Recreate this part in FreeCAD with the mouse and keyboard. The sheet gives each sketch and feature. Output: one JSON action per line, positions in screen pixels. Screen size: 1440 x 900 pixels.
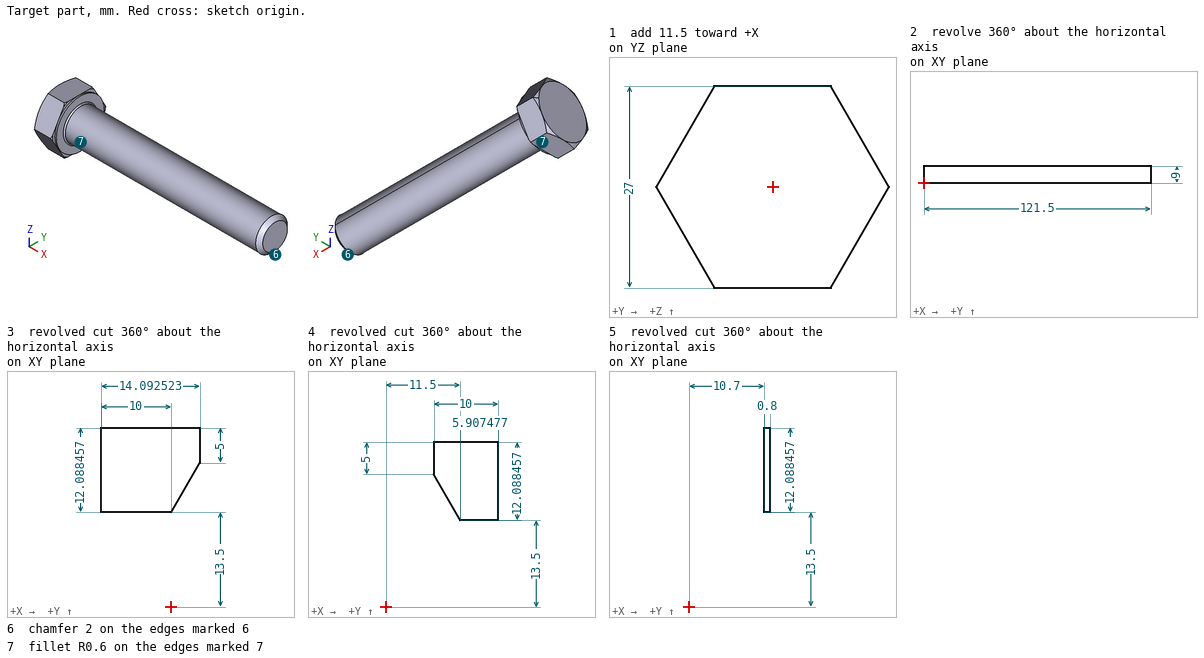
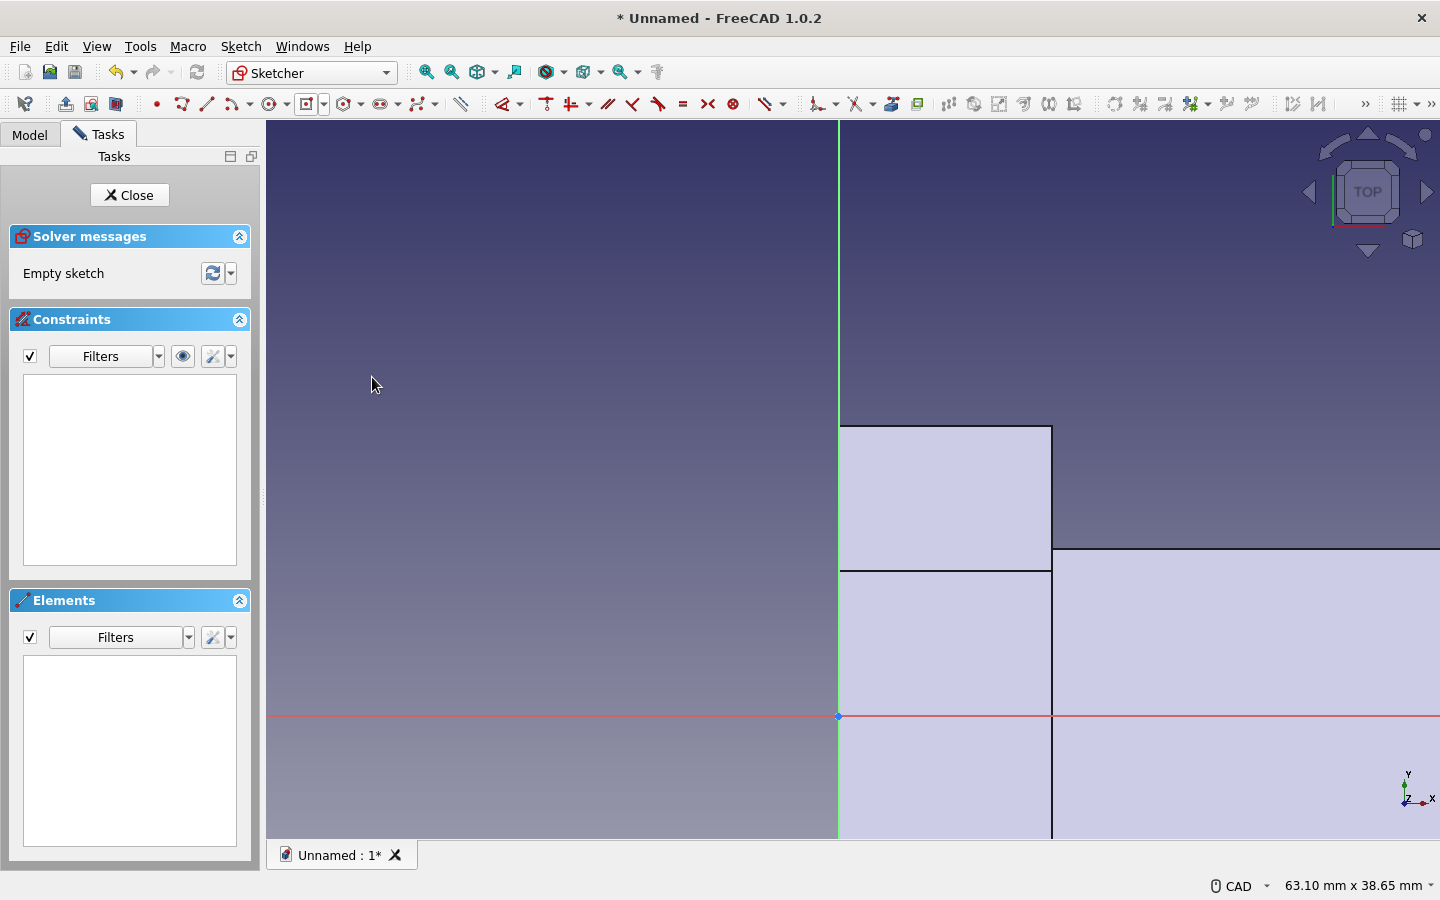
{"action": "key", "text": "g m"}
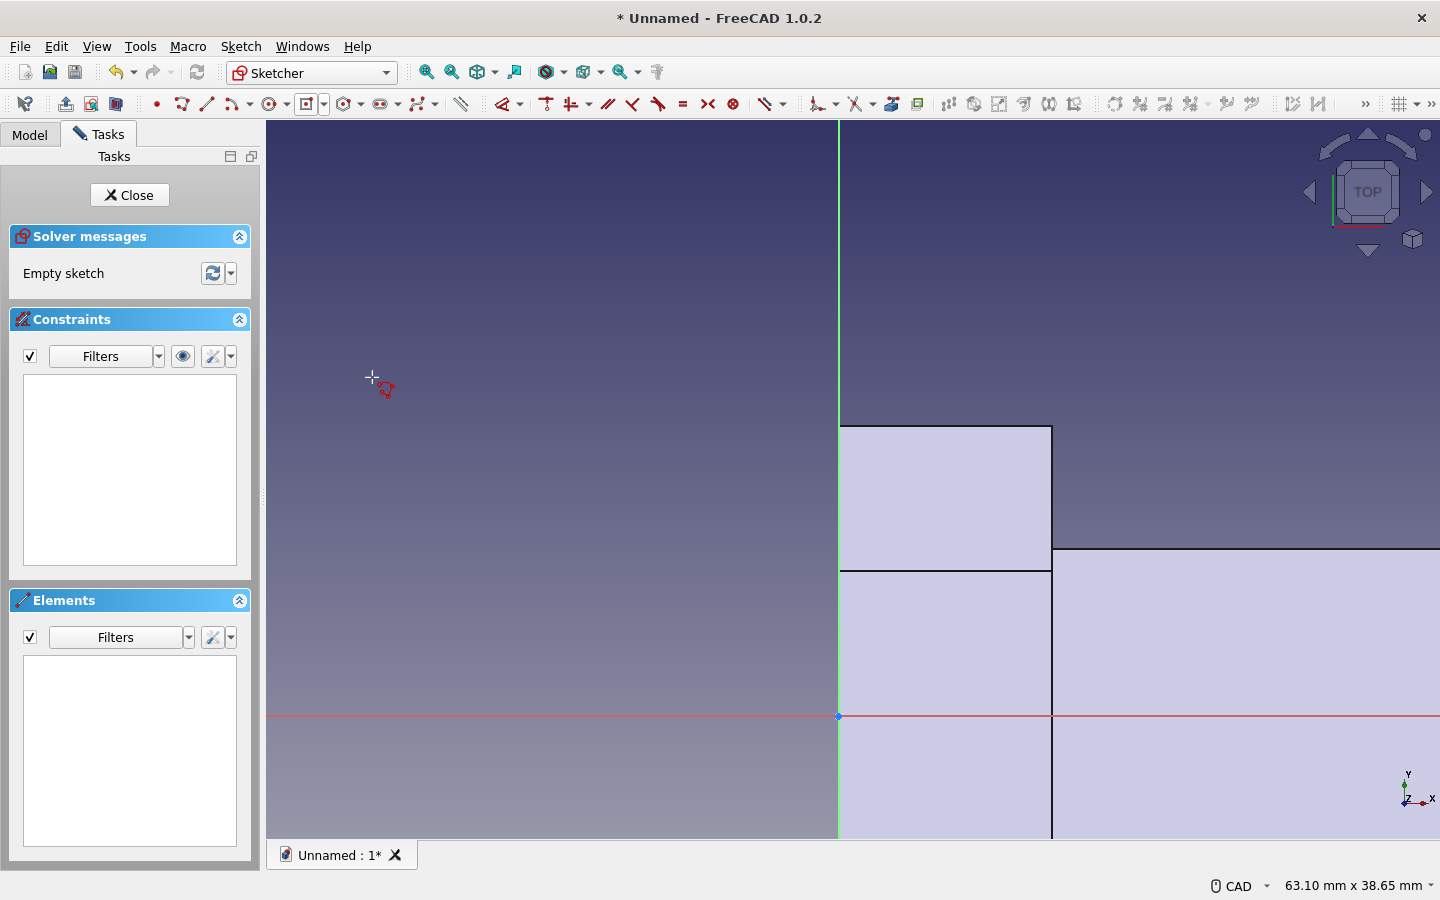
{"action": "left_click", "coordinate": [839, 465]}
{"action": "left_click", "coordinate": [915, 333]}
{"action": "left_click", "coordinate": [915, 240]}
{"action": "left_click", "coordinate": [652, 240]}
{"action": "left_click", "coordinate": [652, 465]}
{"action": "left_click", "coordinate": [839, 466]}
{"action": "key", "text": "Escape"}
{"action": "key", "text": "Escape"}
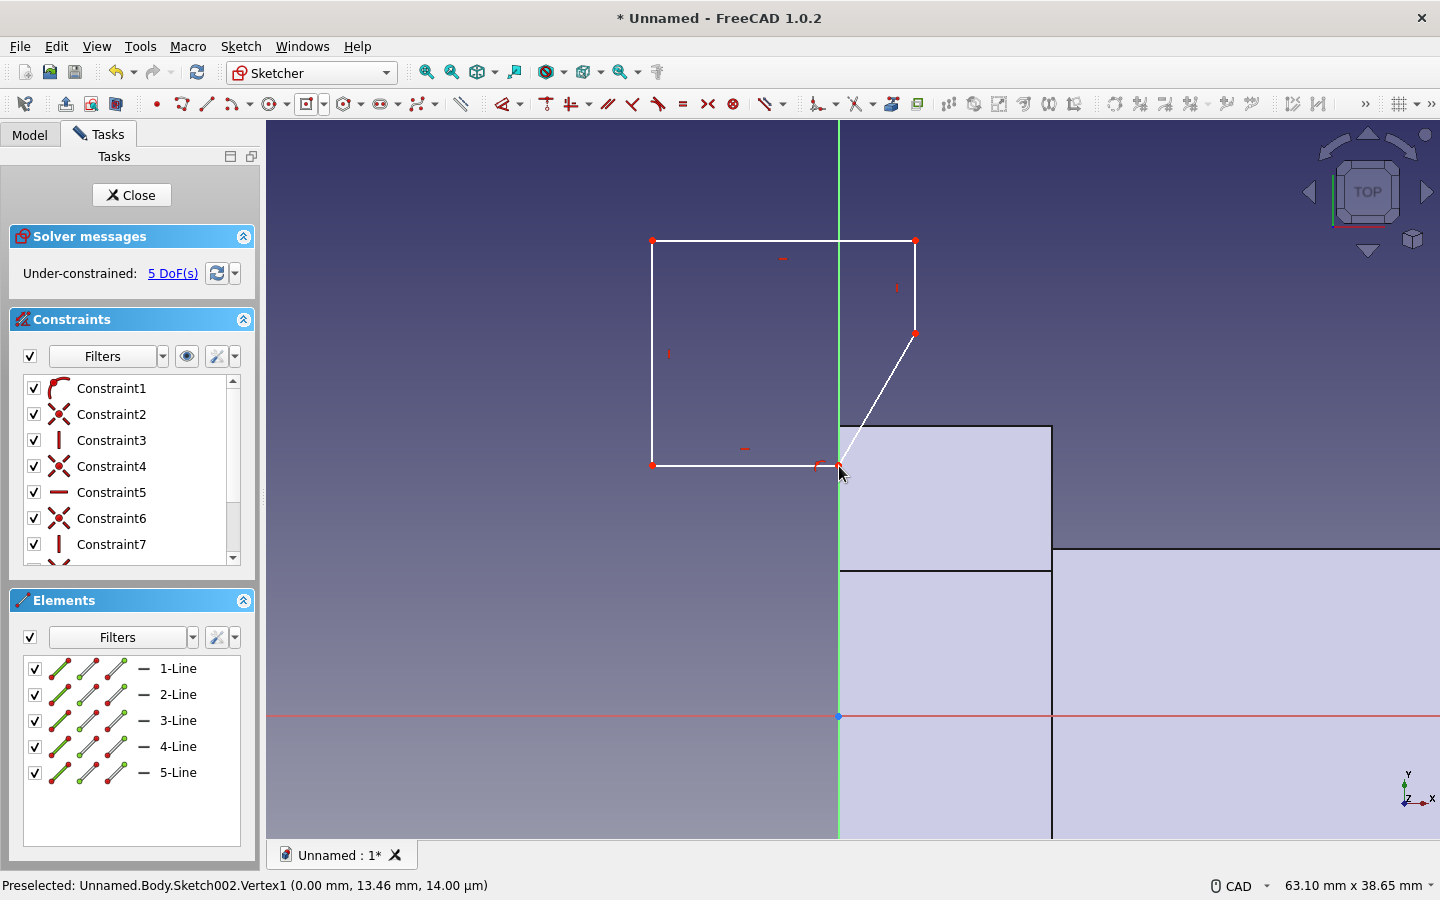
{"action": "left_click", "coordinate": [502, 104]}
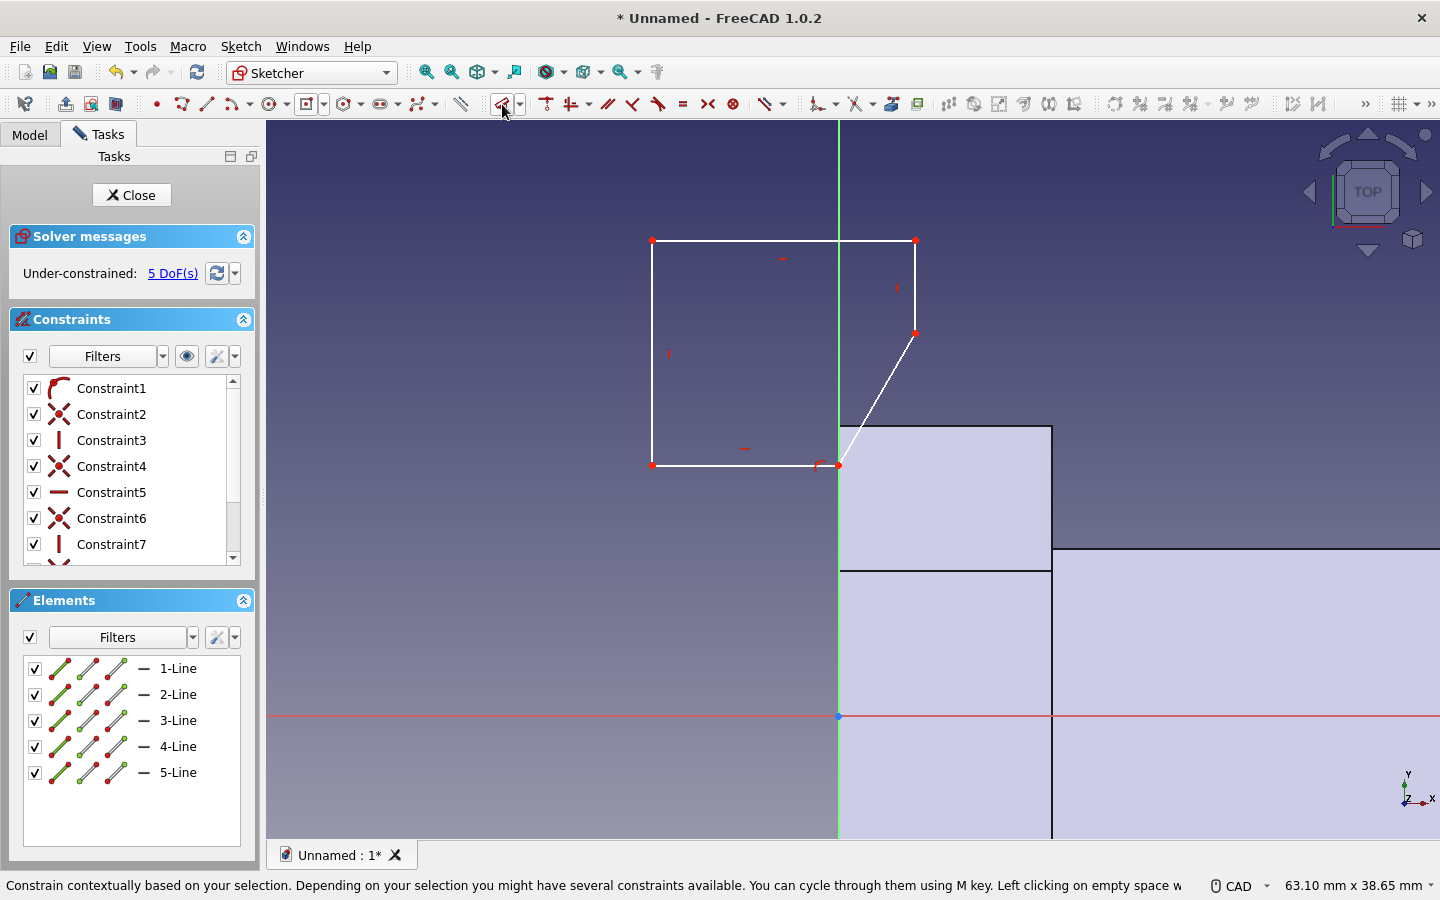
{"action": "left_click", "coordinate": [915, 306]}
{"action": "left_click", "coordinate": [949, 288]}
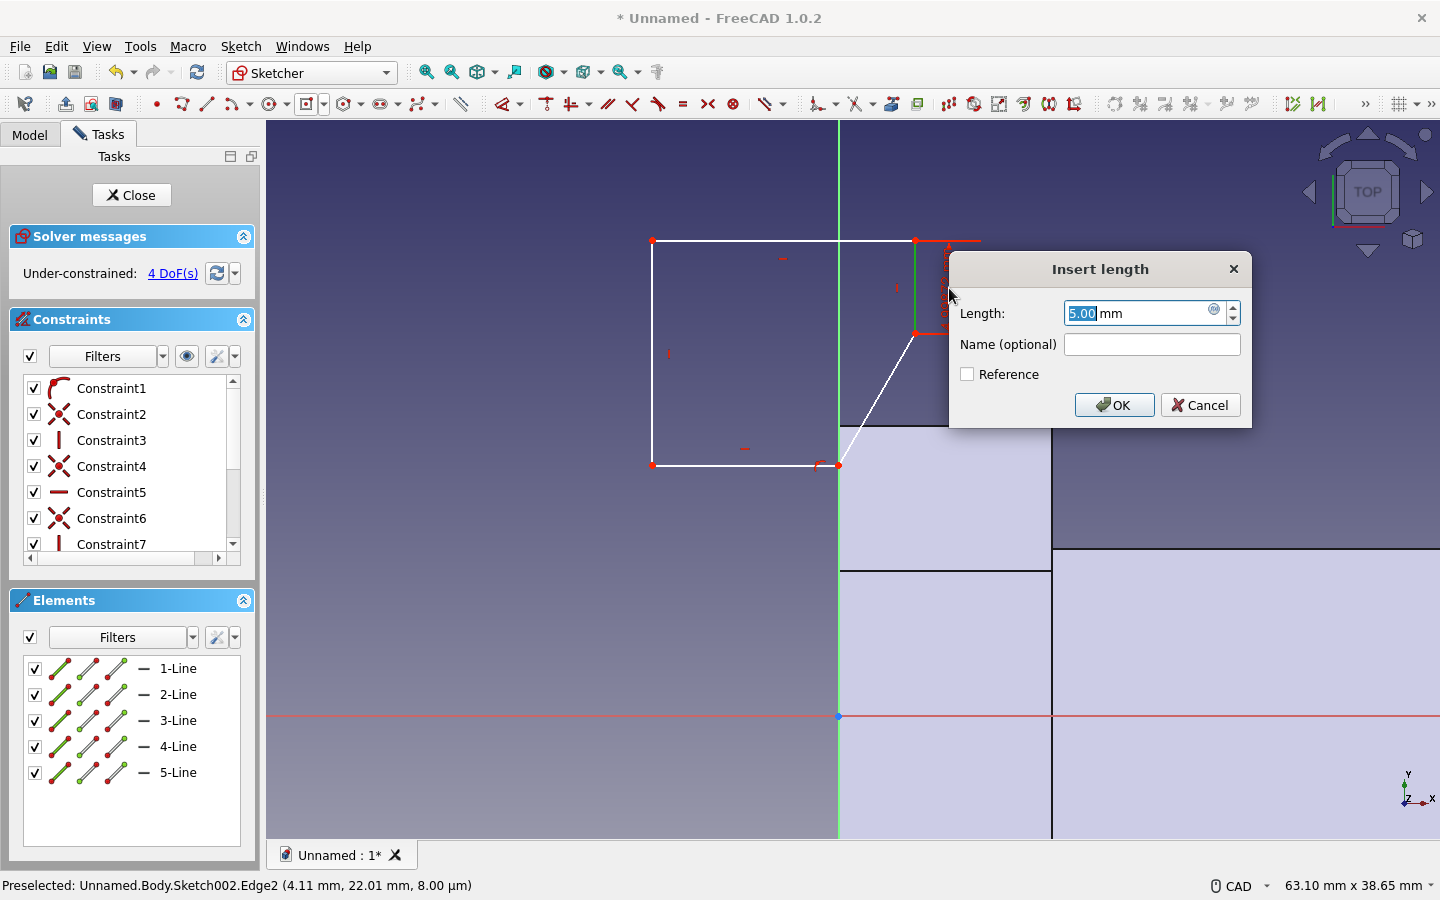
{"action": "type", "text": "5"}
{"action": "key", "text": "Return"}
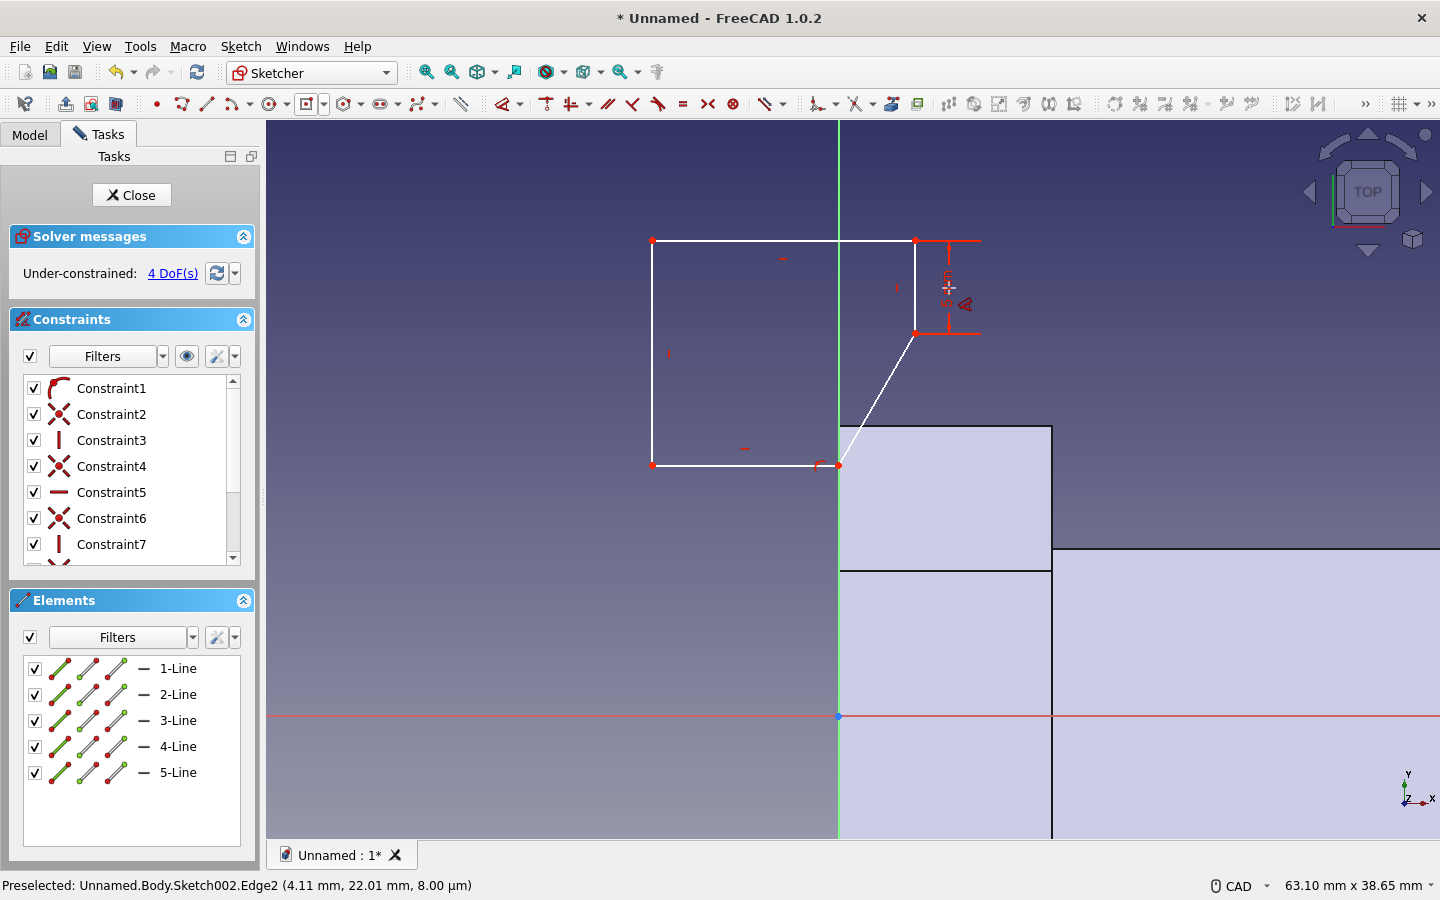
{"action": "left_click", "coordinate": [708, 466]}
{"action": "left_click", "coordinate": [745, 432]}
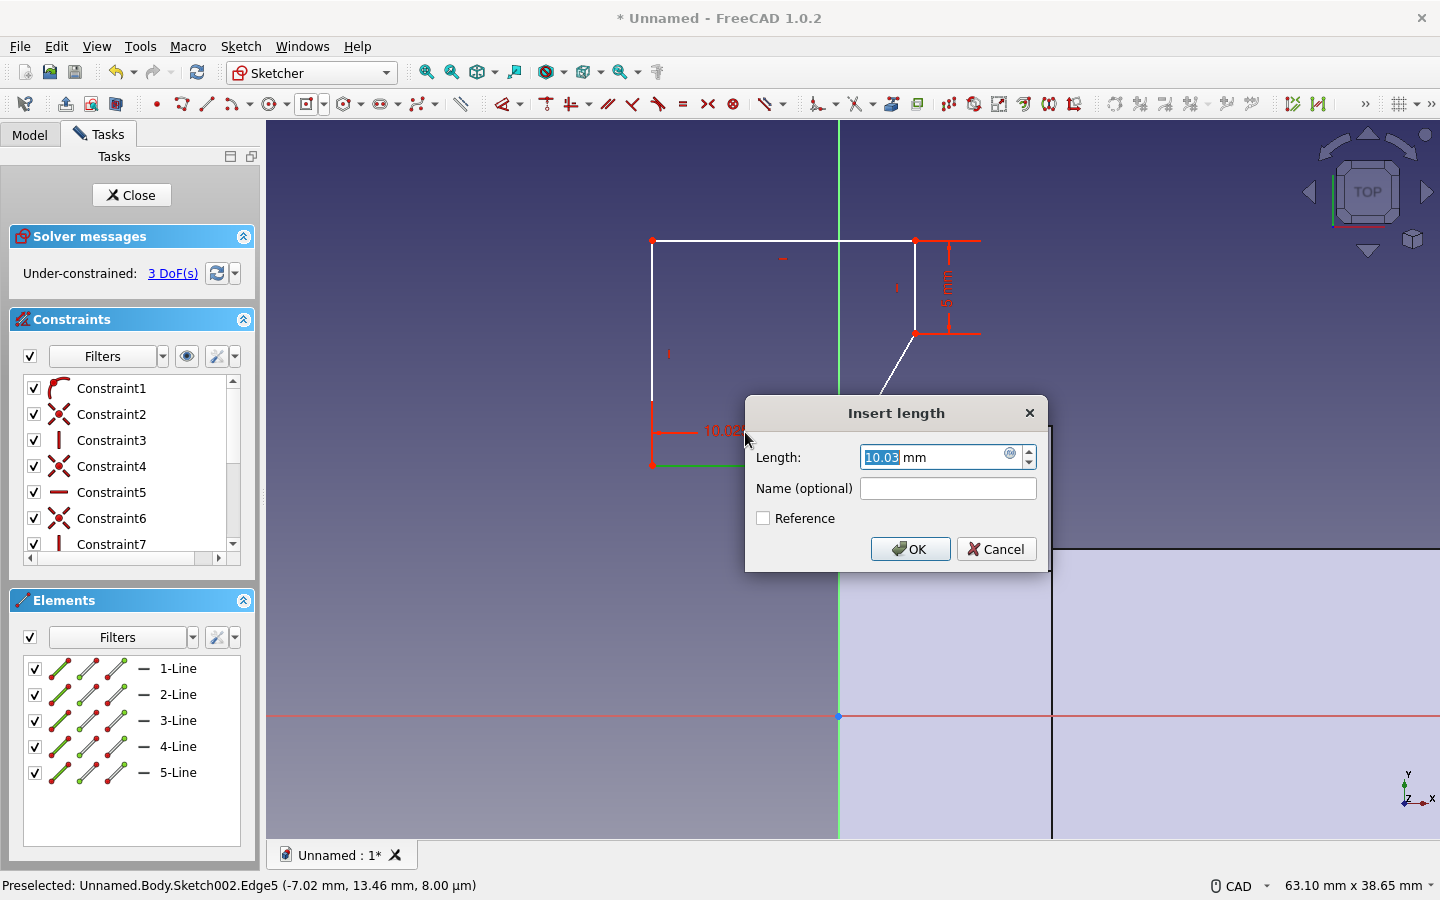
{"action": "type", "text": "10"}
{"action": "key", "text": "Return"}